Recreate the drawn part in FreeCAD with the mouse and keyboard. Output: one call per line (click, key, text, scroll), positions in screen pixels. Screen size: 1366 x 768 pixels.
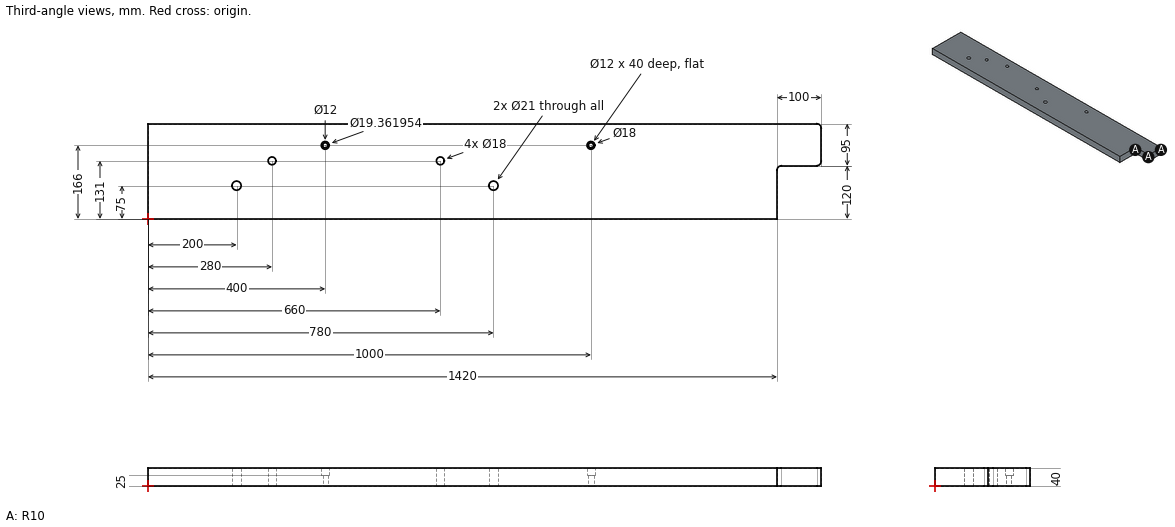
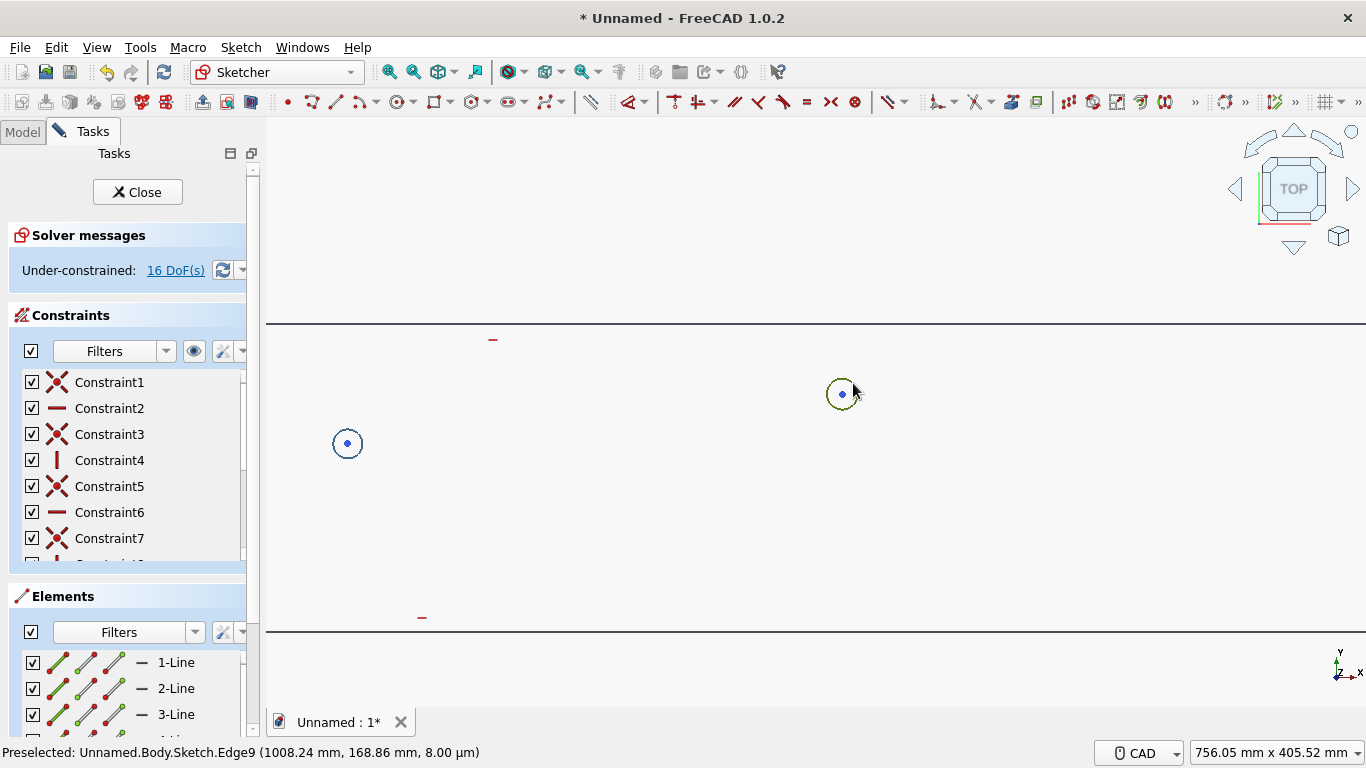
scroll(856, 384, down, 6)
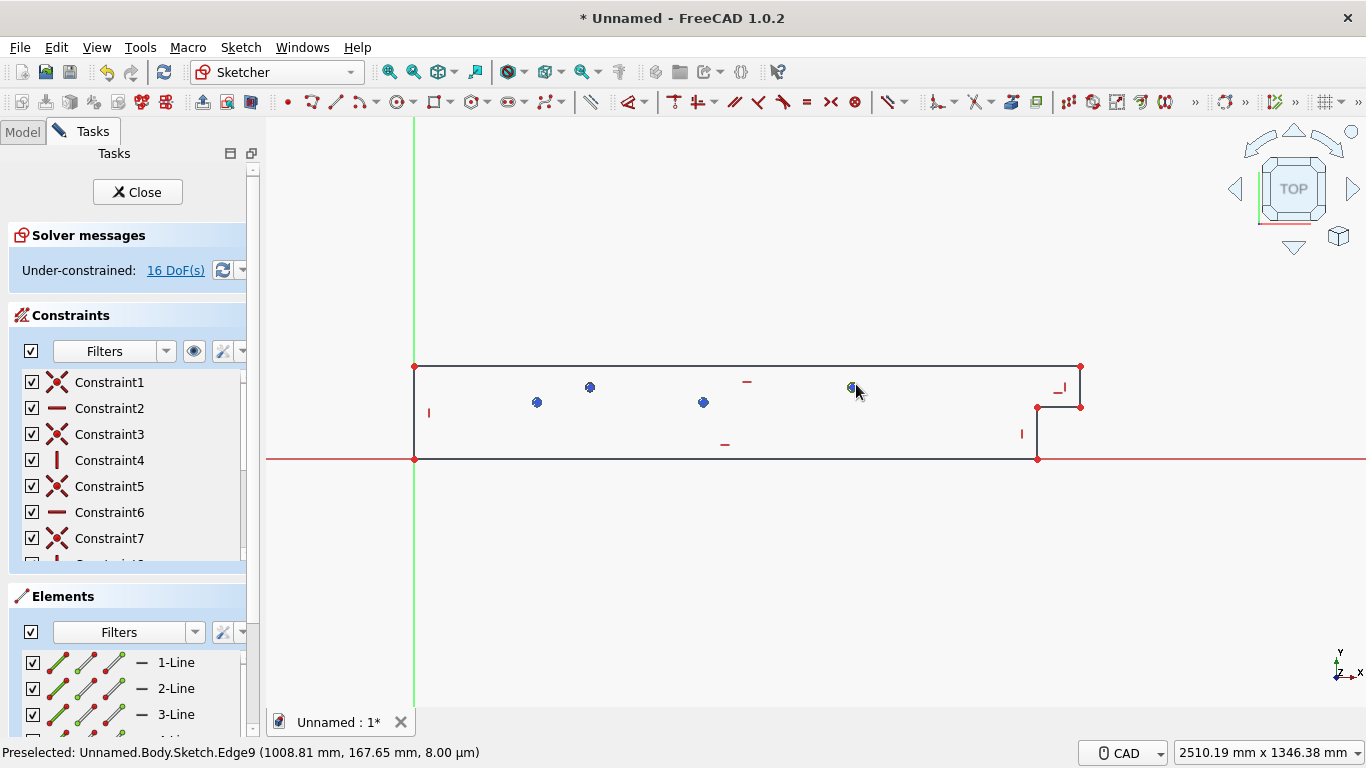
scroll(593, 384, up, 6)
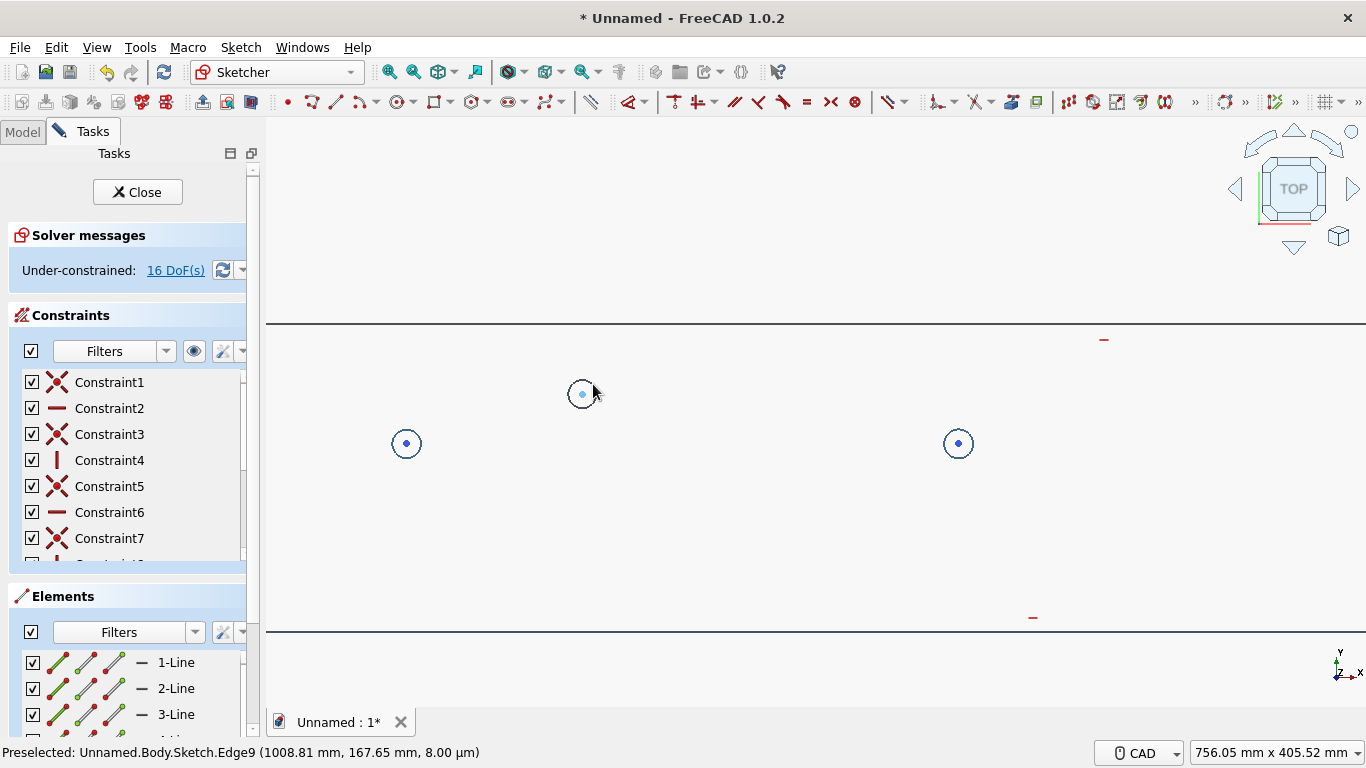
click(592, 384)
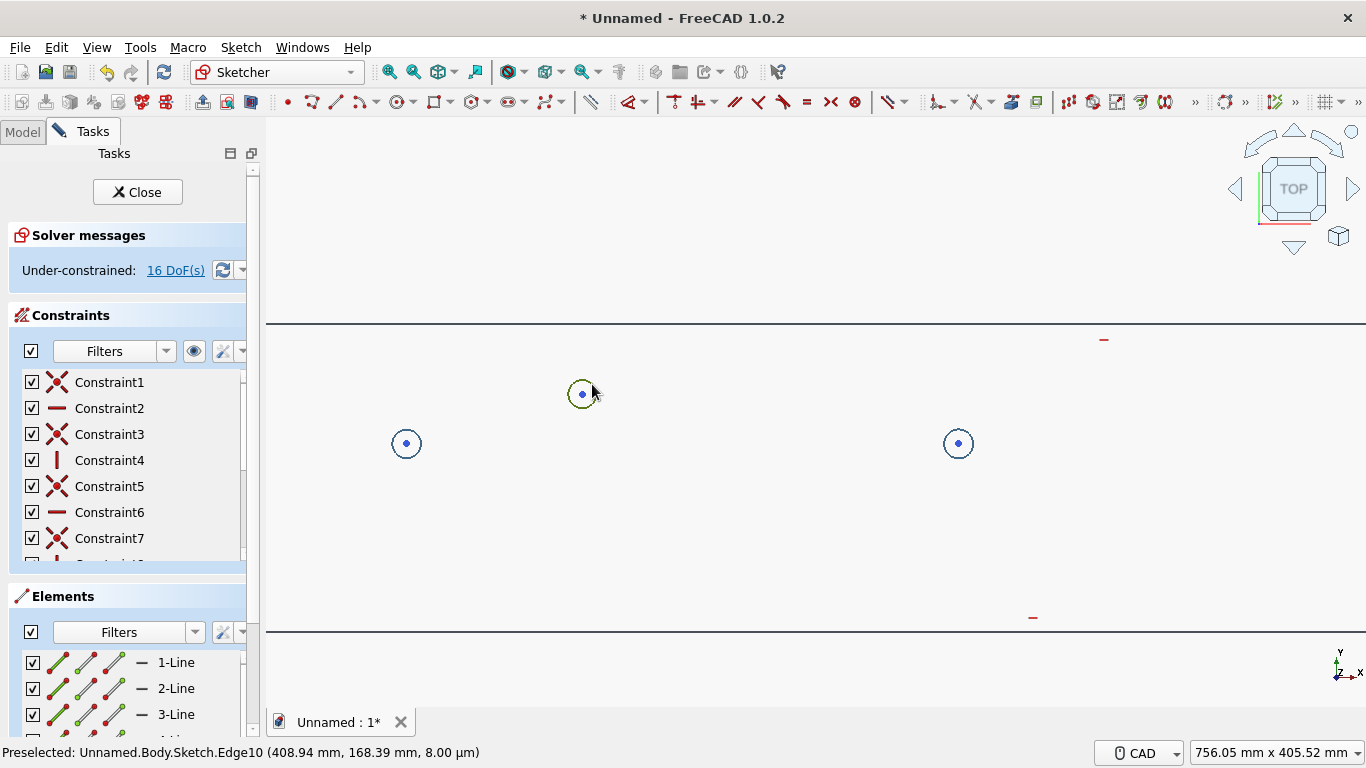
key(e)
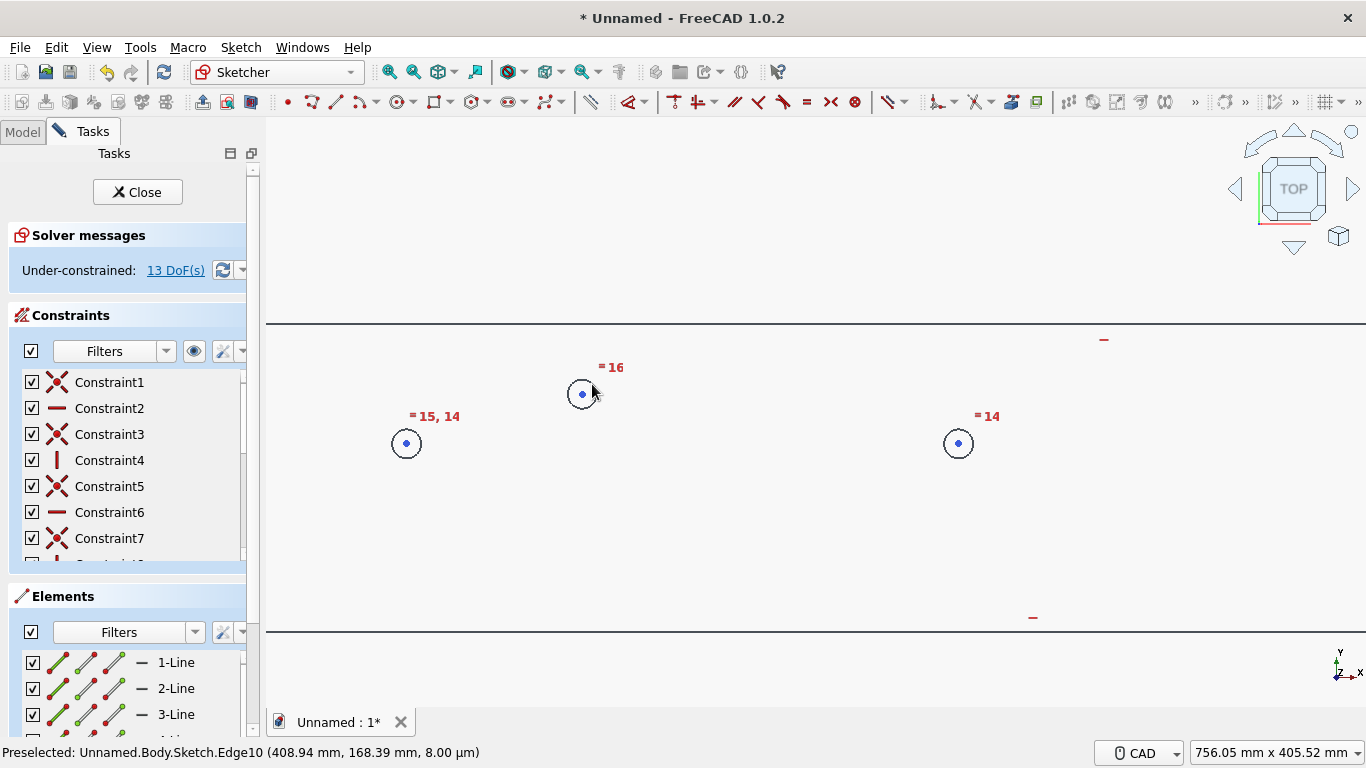
key(d)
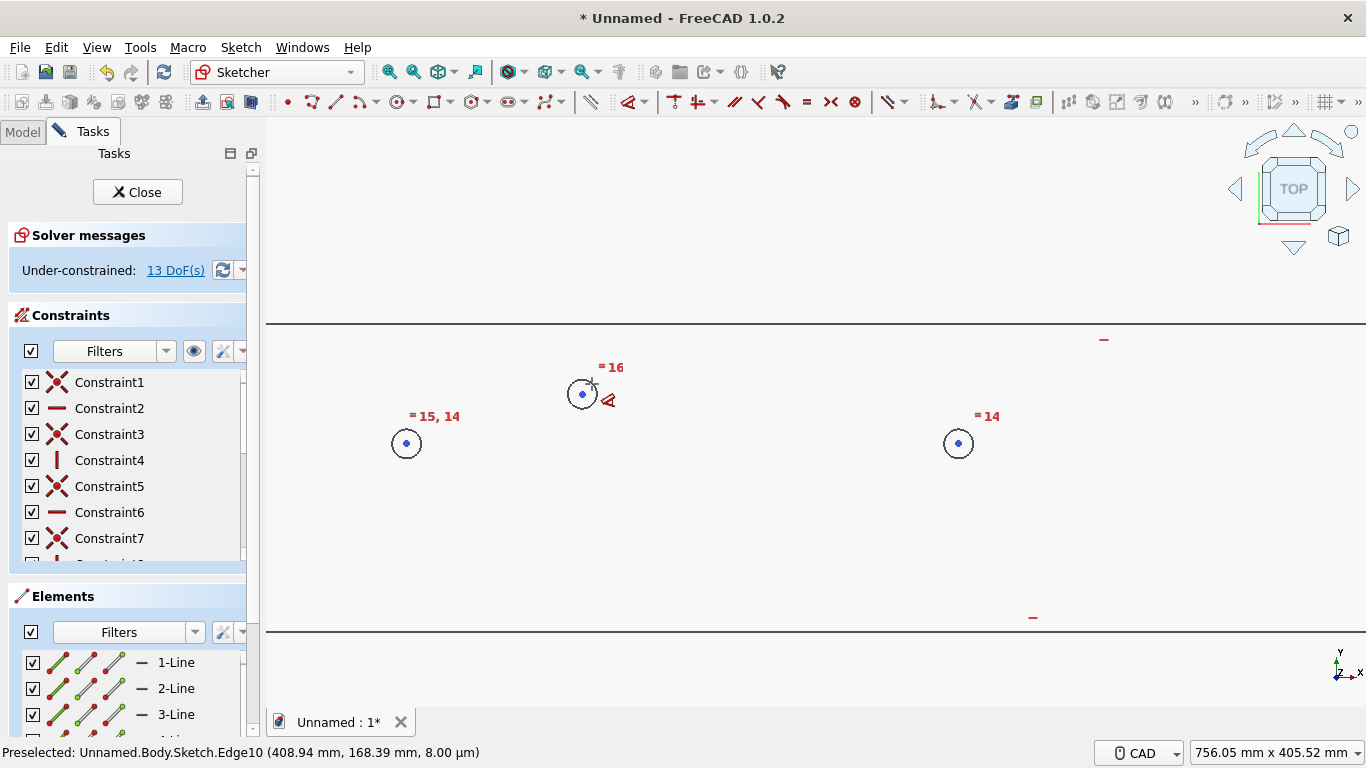
scroll(969, 434, up, 3)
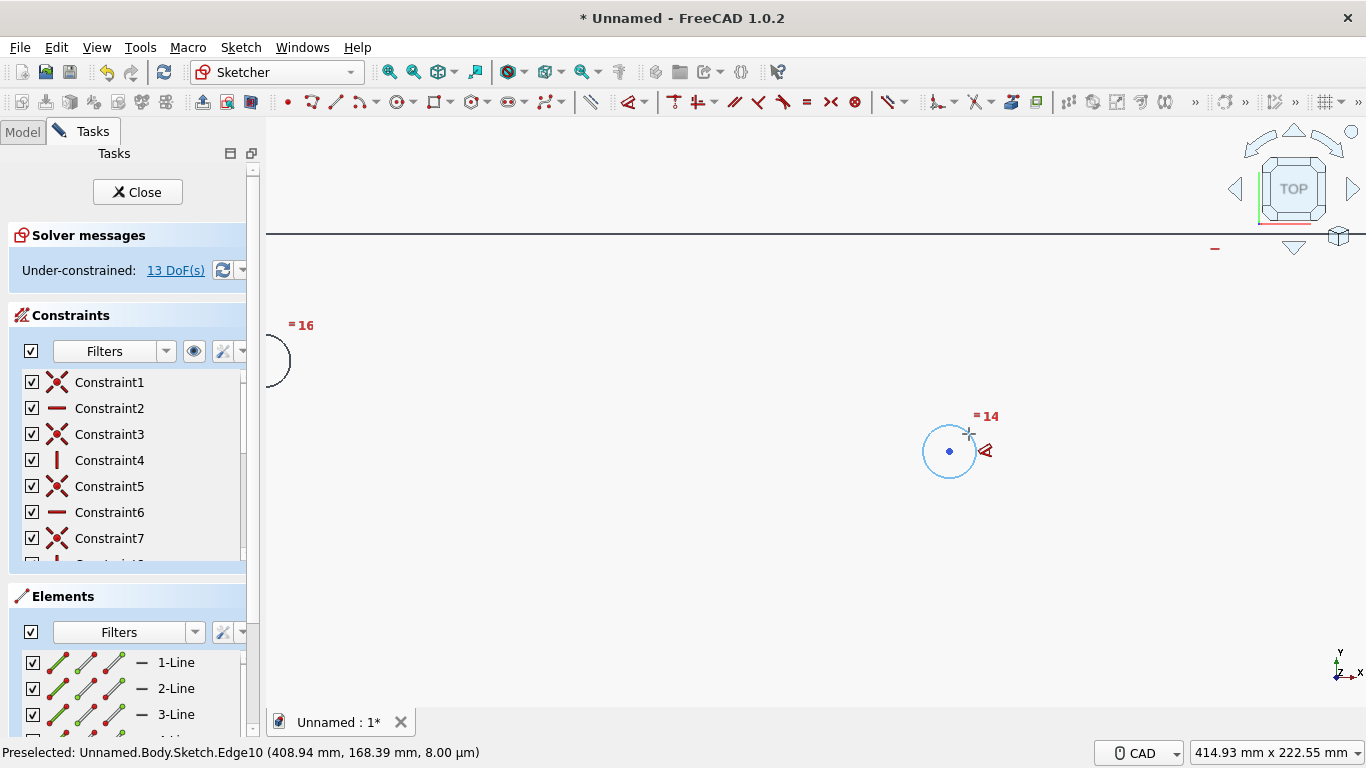
click(968, 433)
click(991, 410)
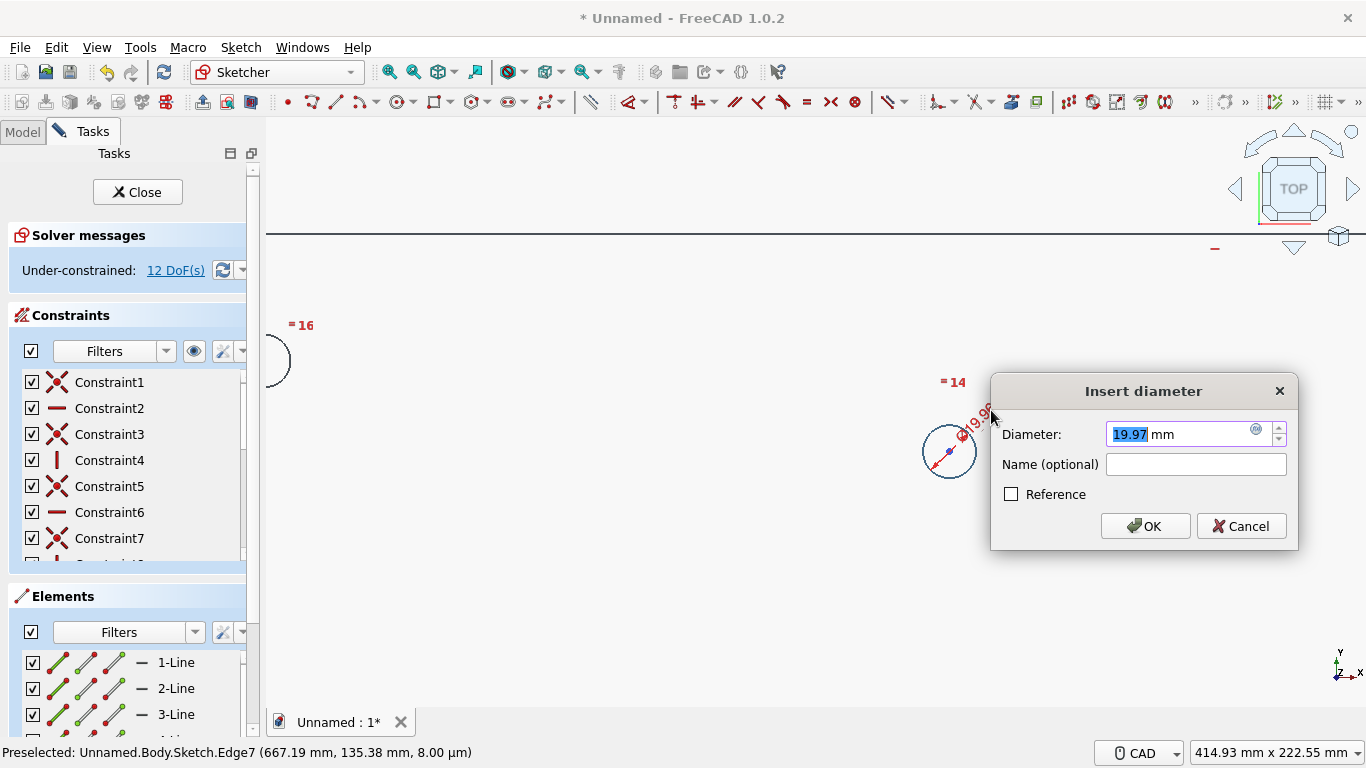
text(18)
key(Return)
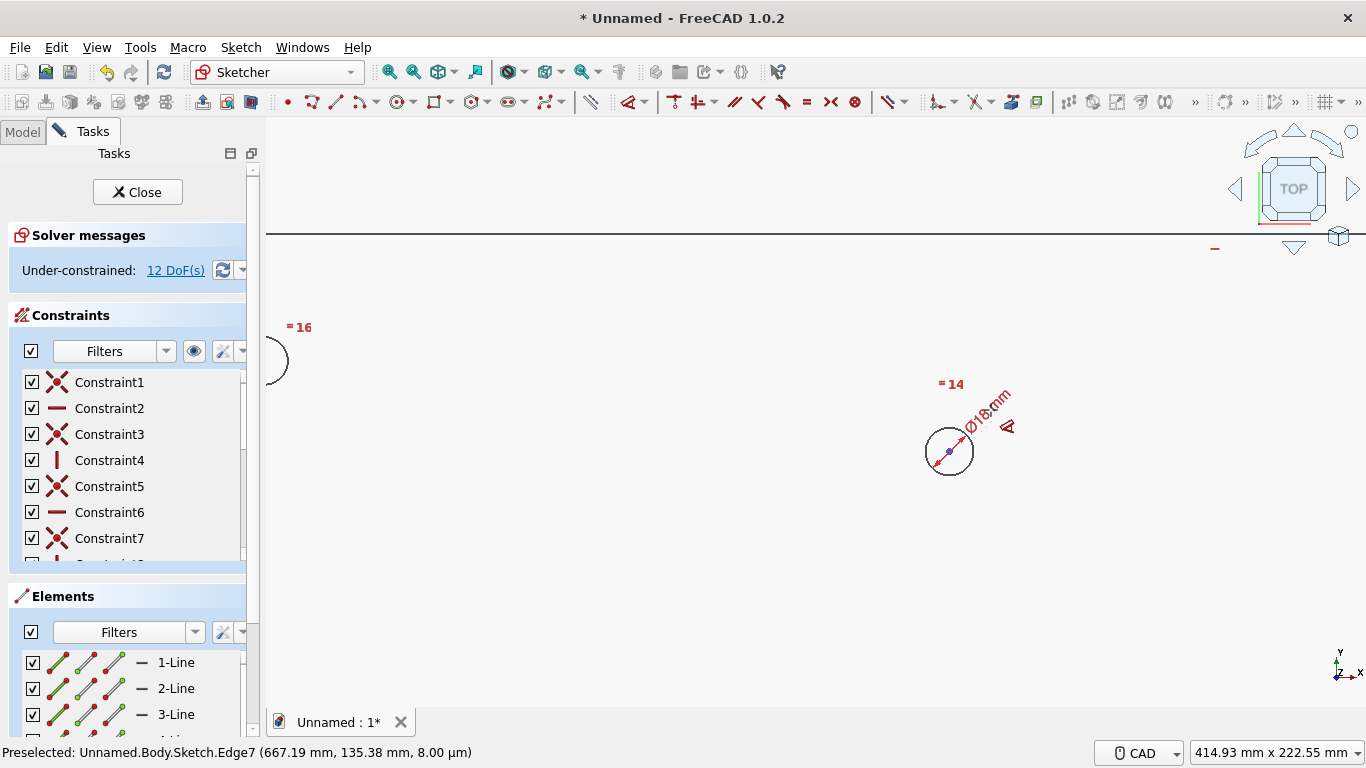
scroll(655, 393, down, 9)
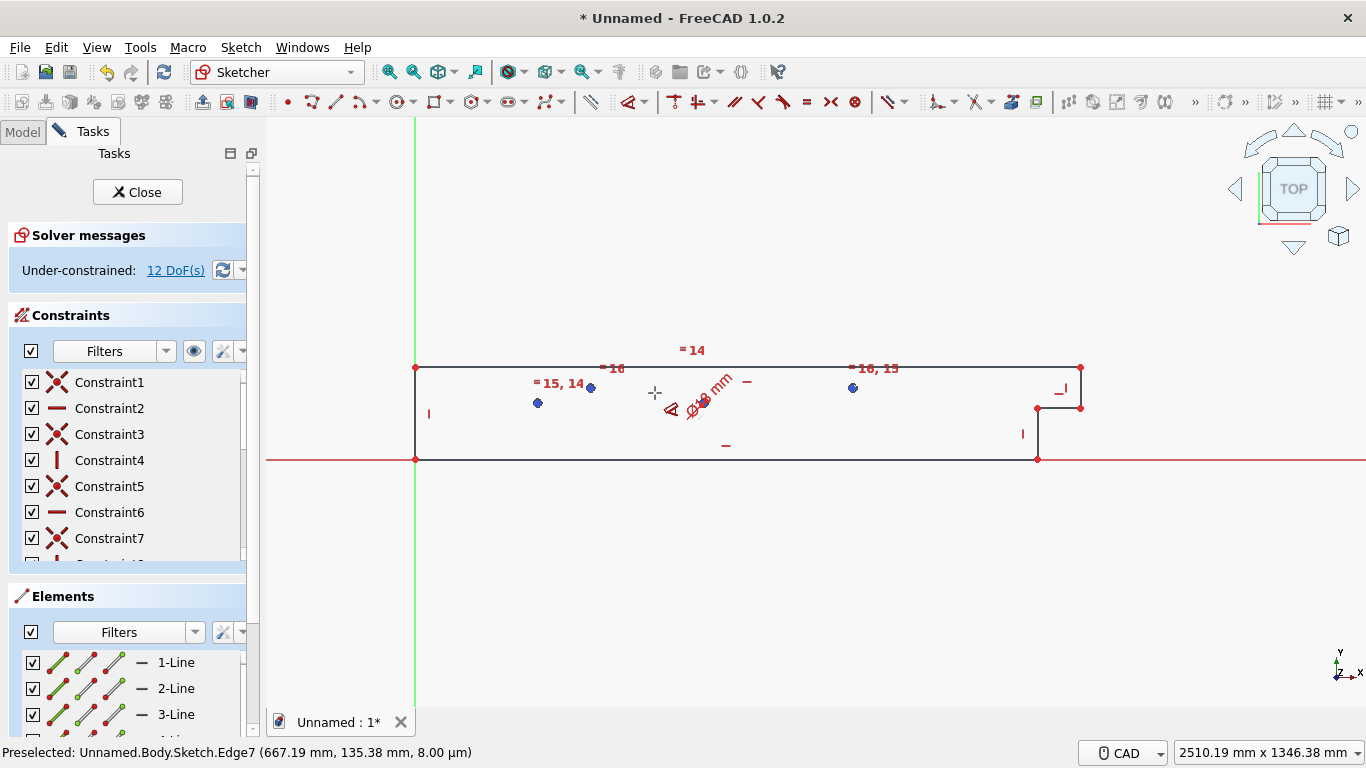
click(1081, 396)
click(1115, 388)